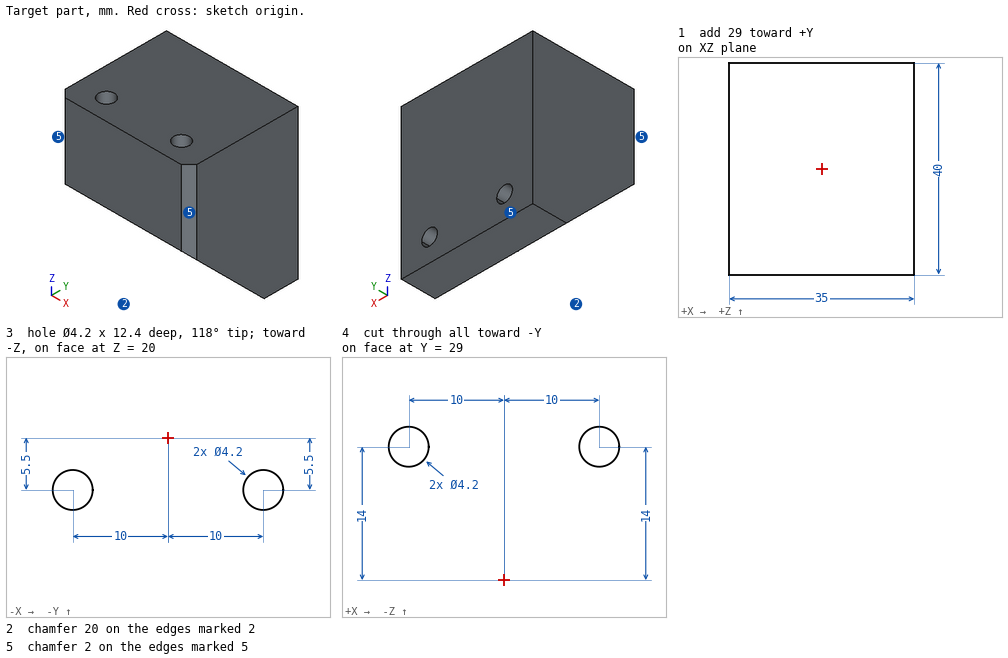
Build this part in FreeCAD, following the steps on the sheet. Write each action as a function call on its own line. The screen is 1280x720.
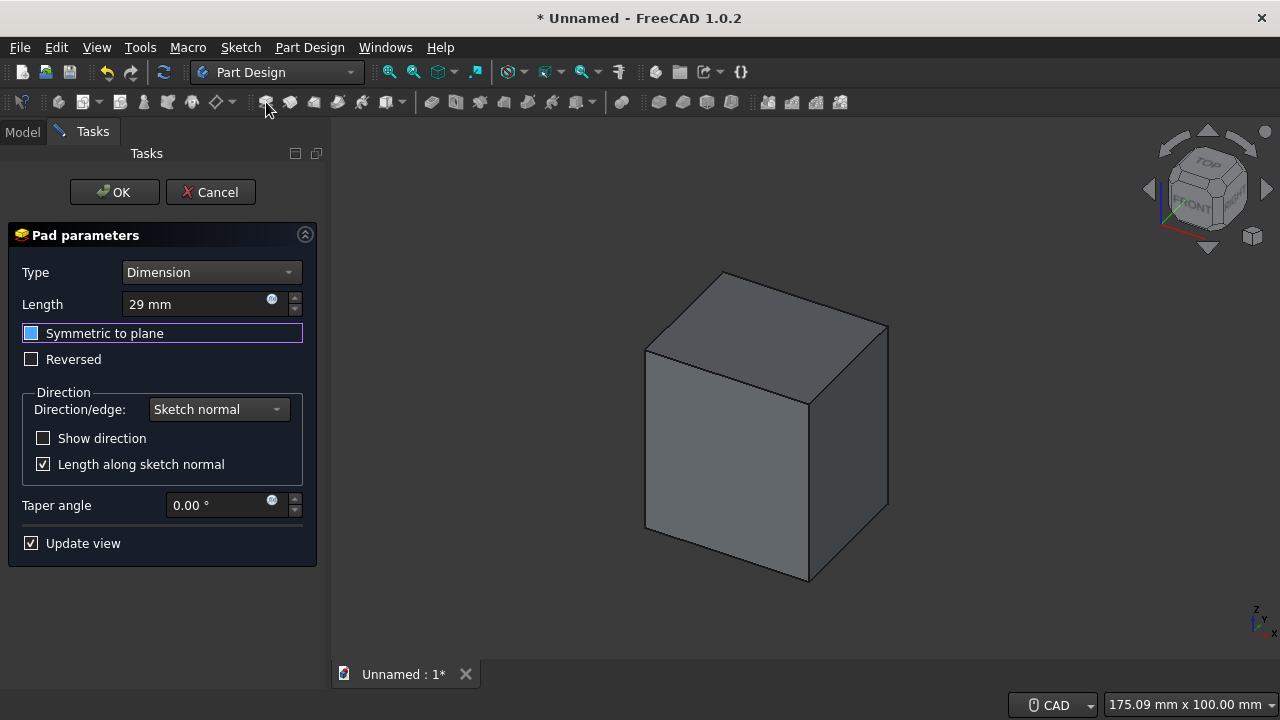
click(30, 359)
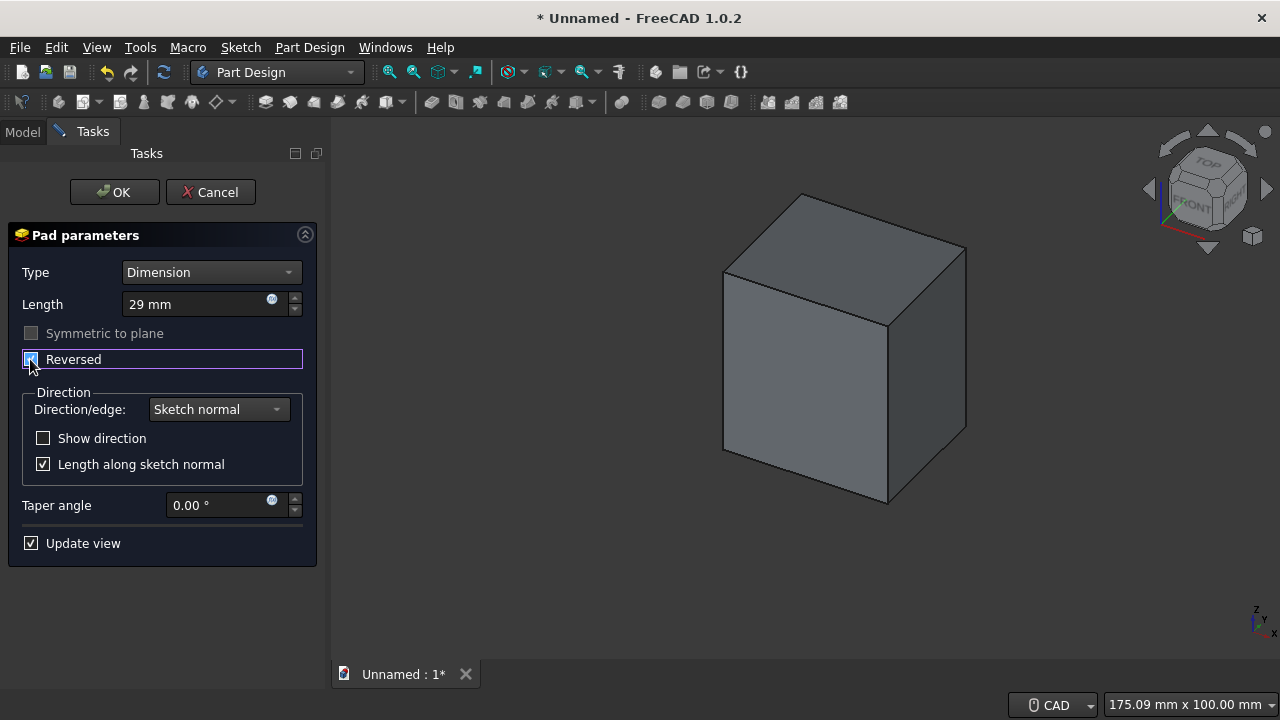
click(115, 192)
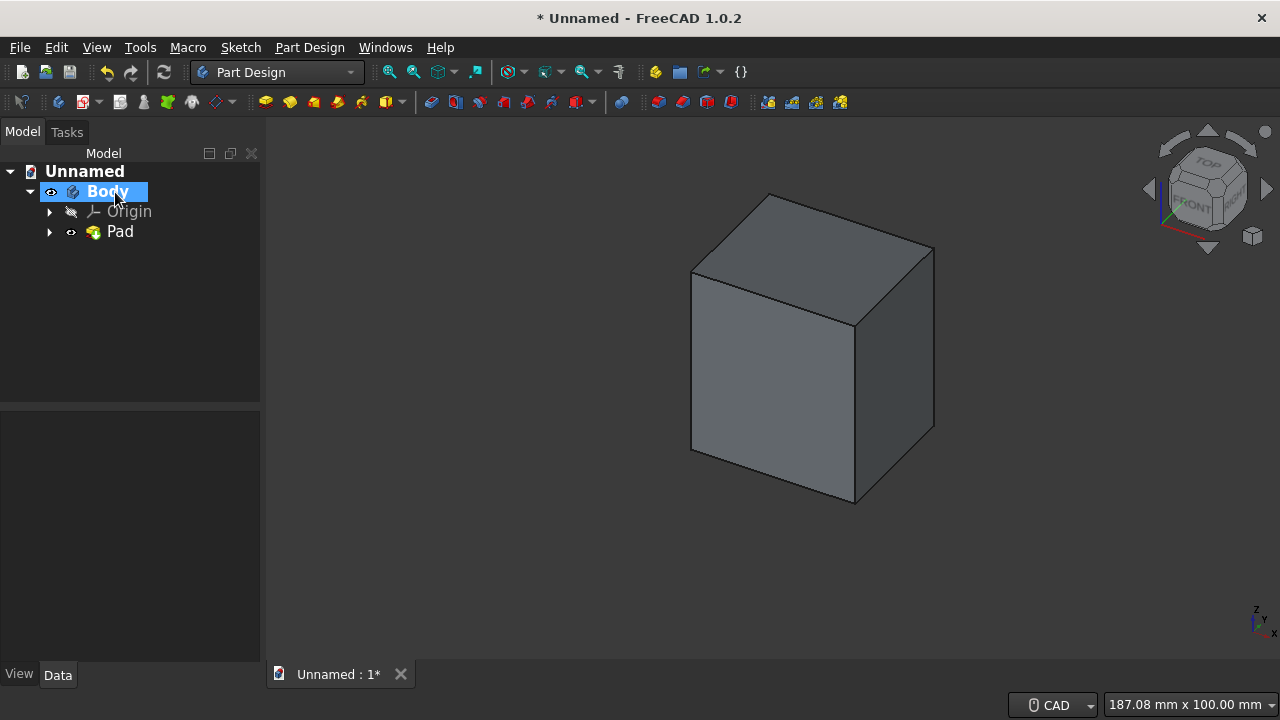
key(0)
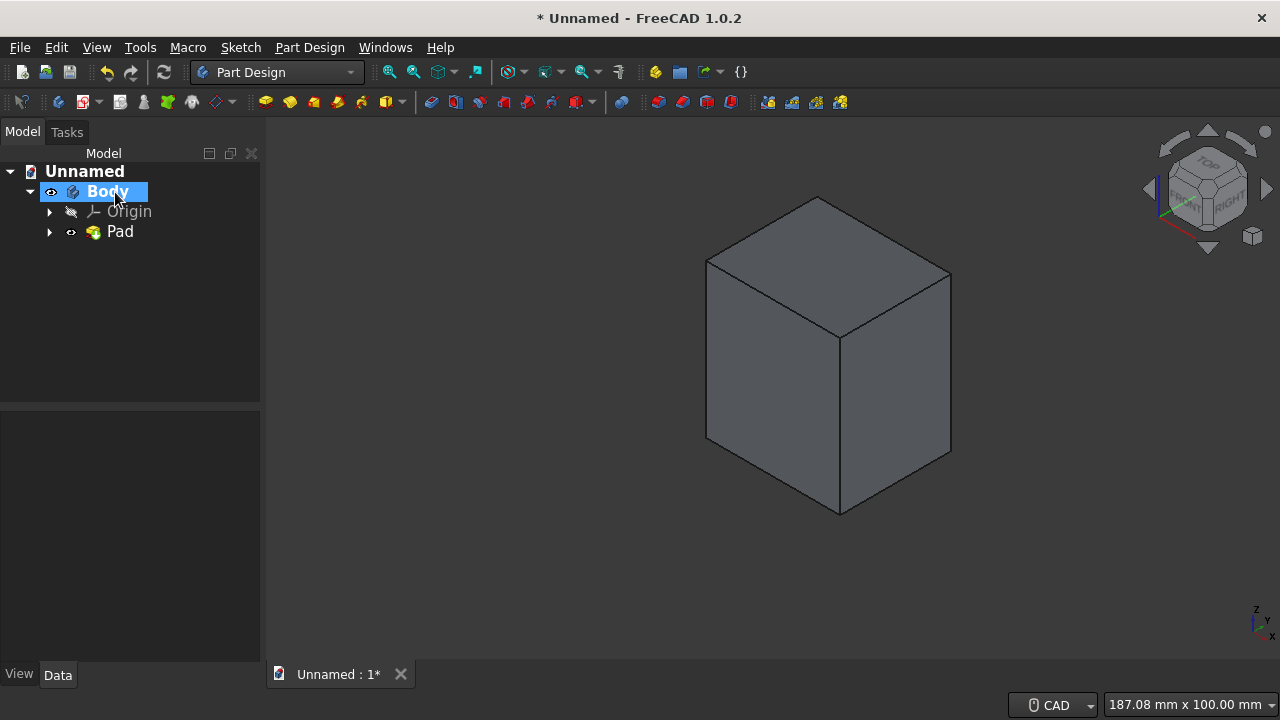
key(2)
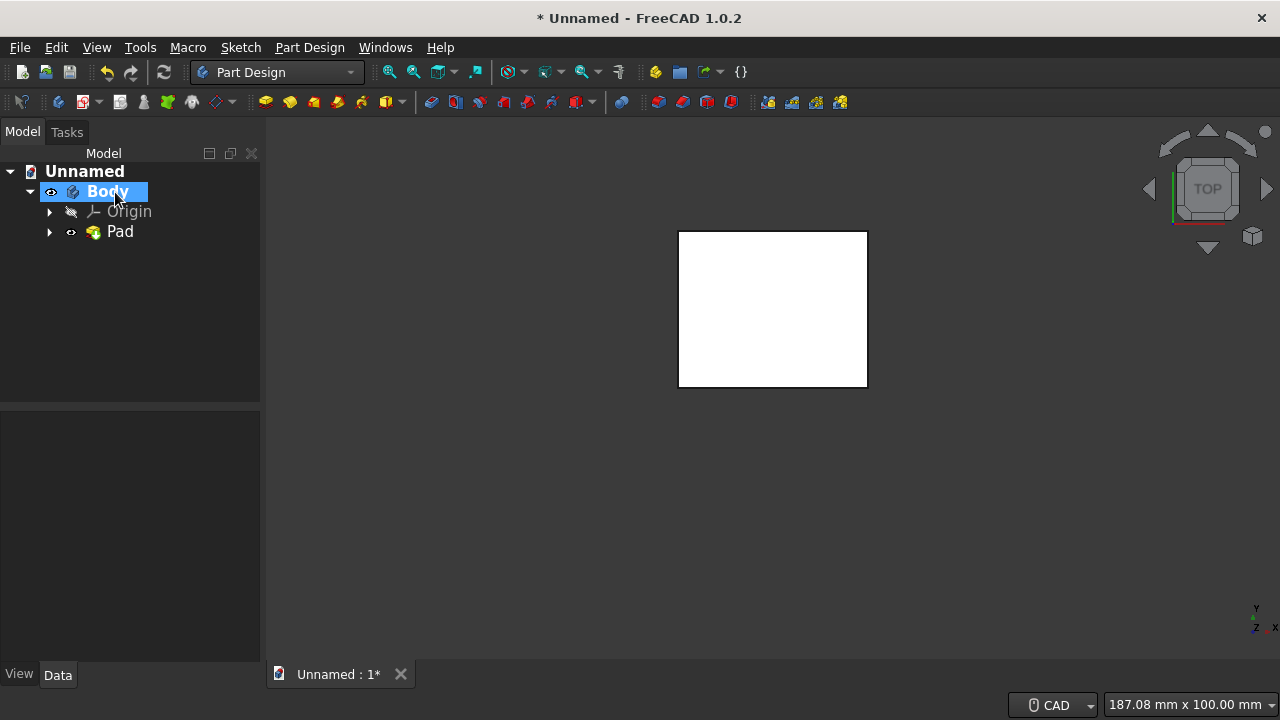
click(390, 72)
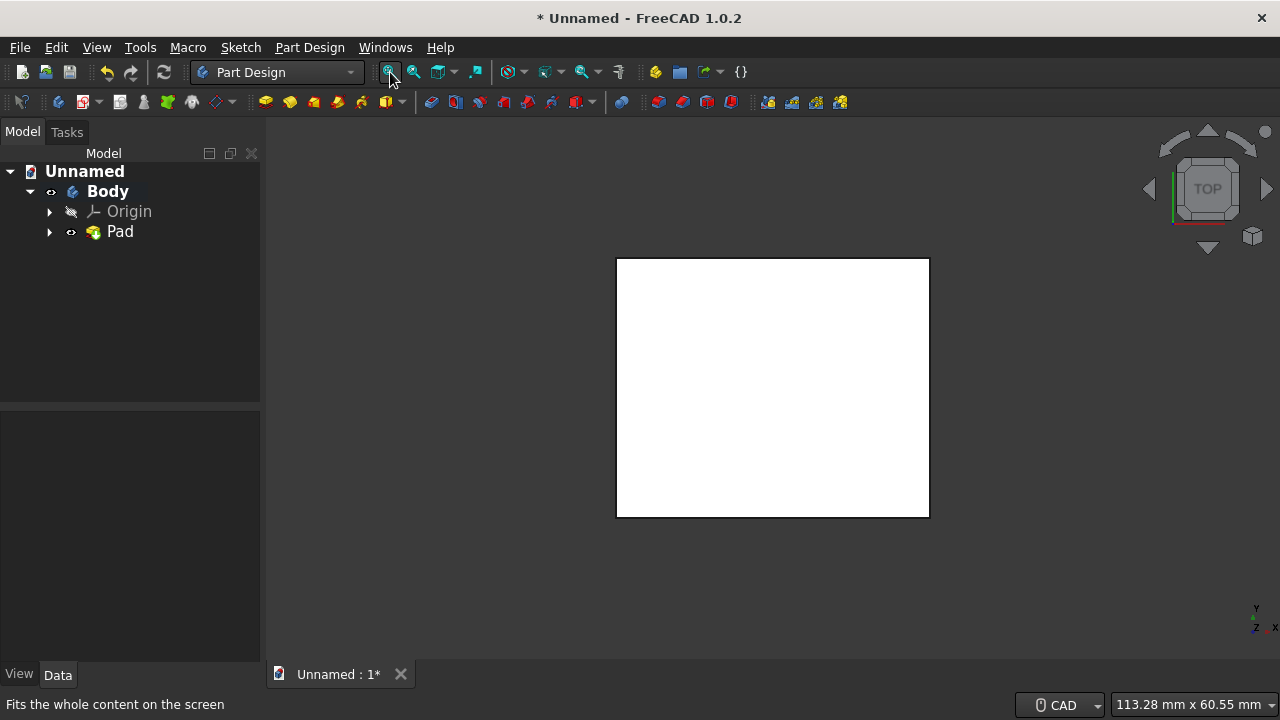
key(1)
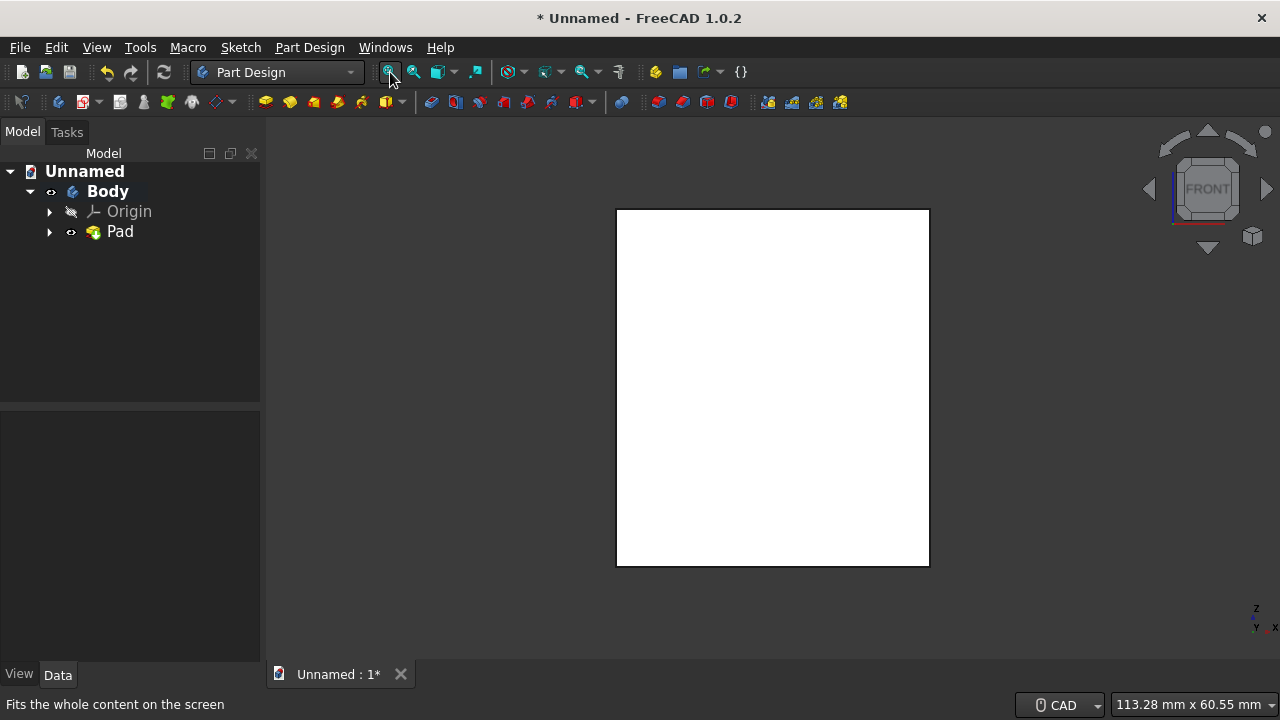
key(3)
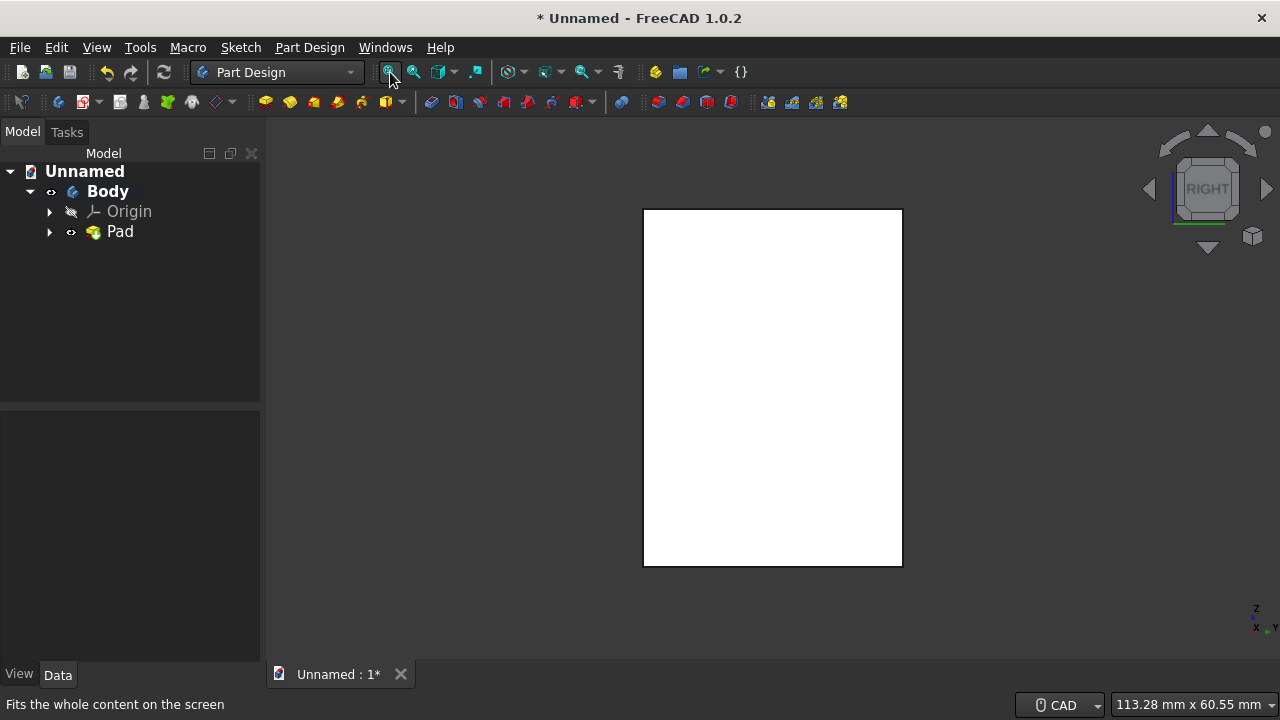
key(5)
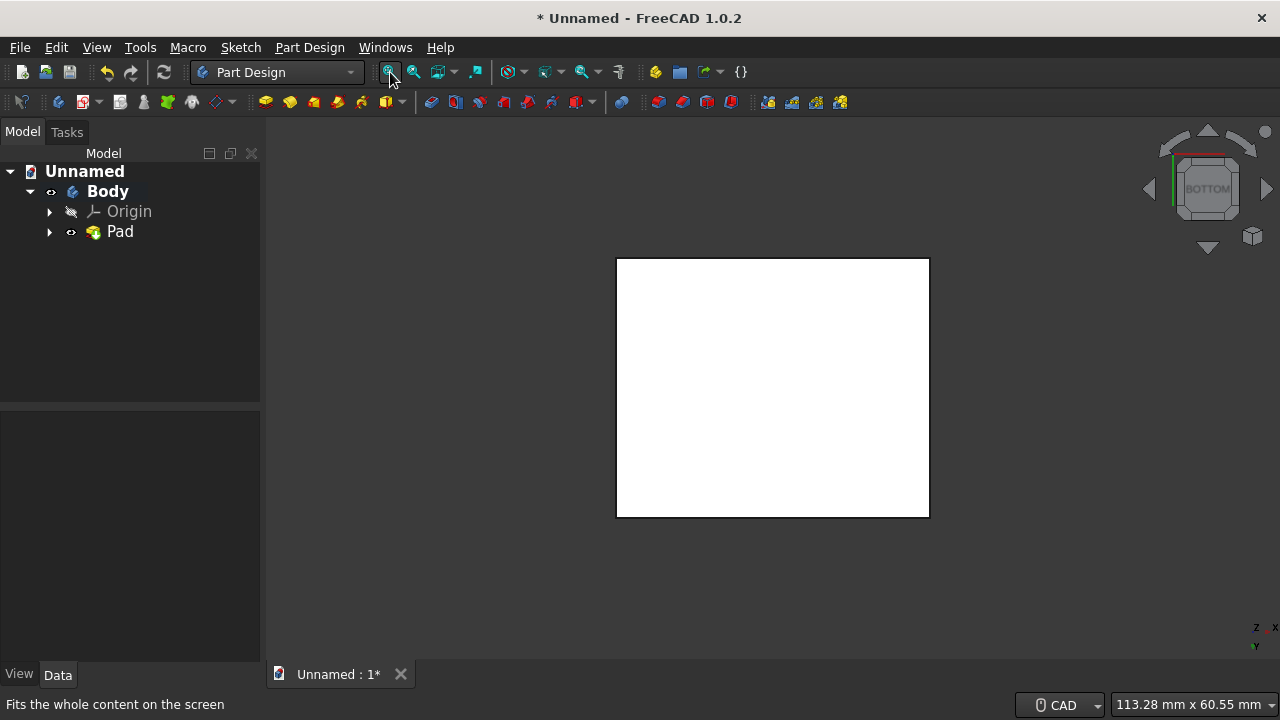
click(773, 257)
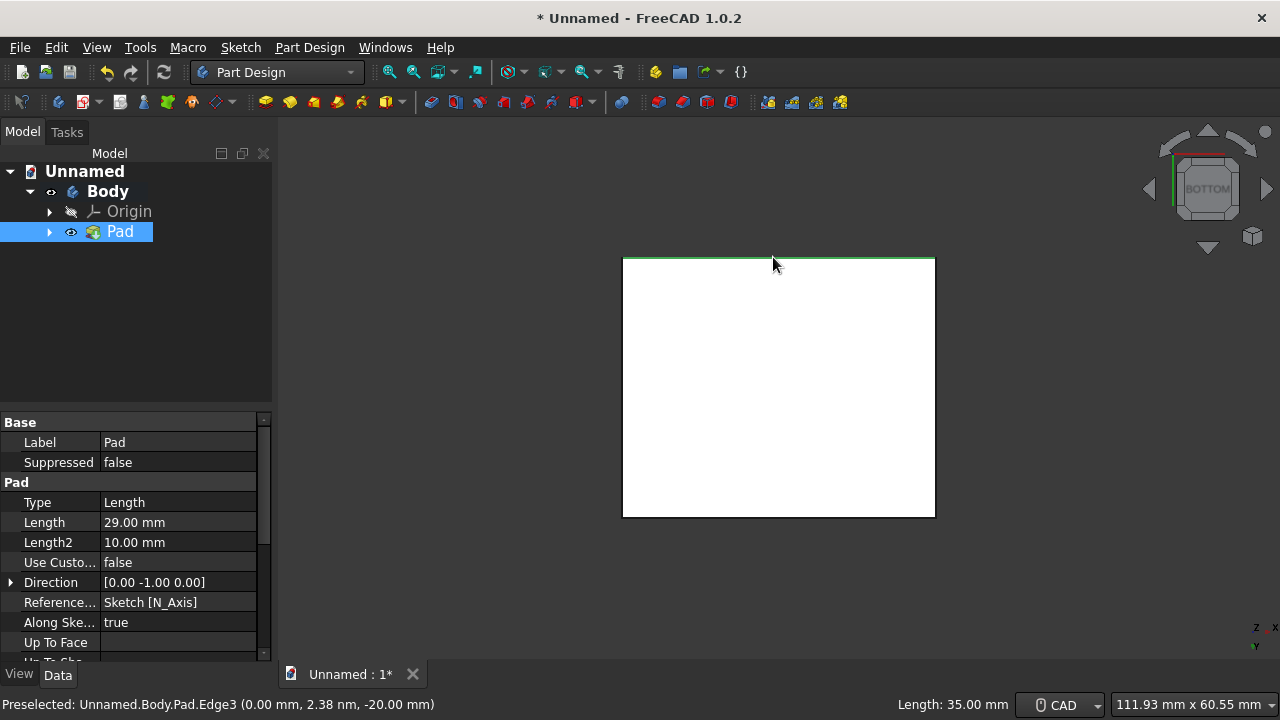
click(684, 102)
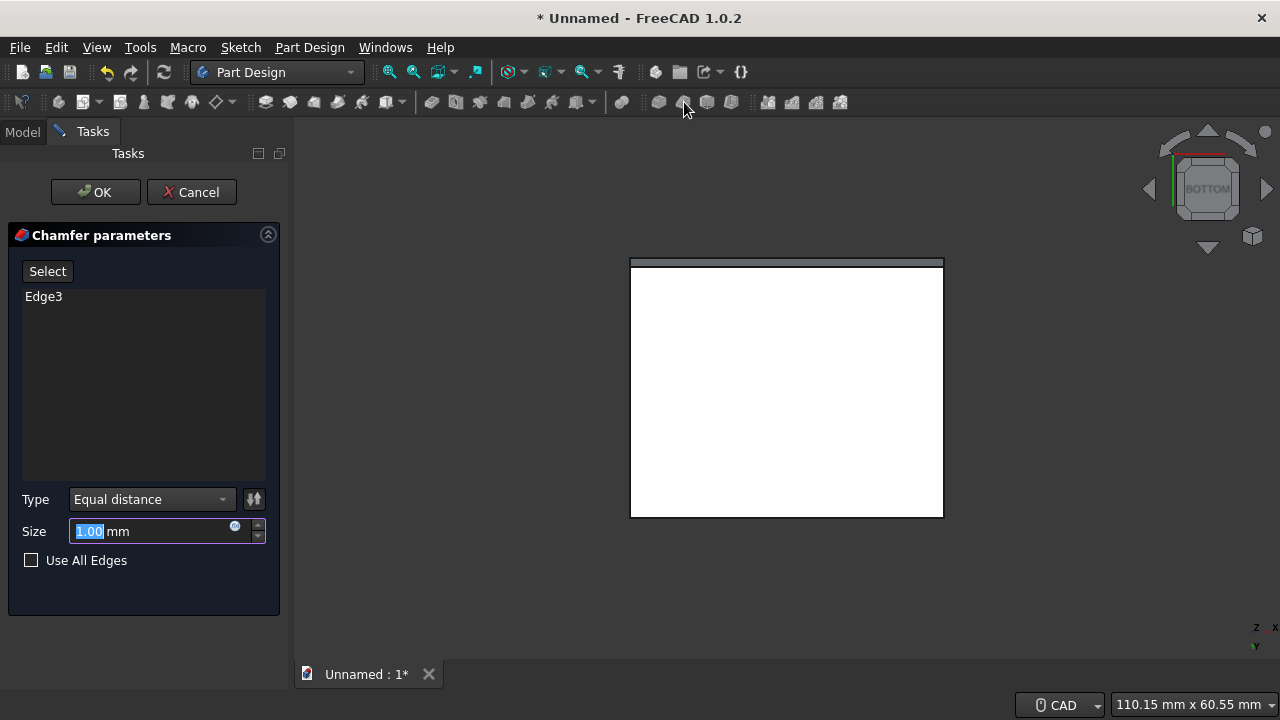
text(20)
key(Tab)